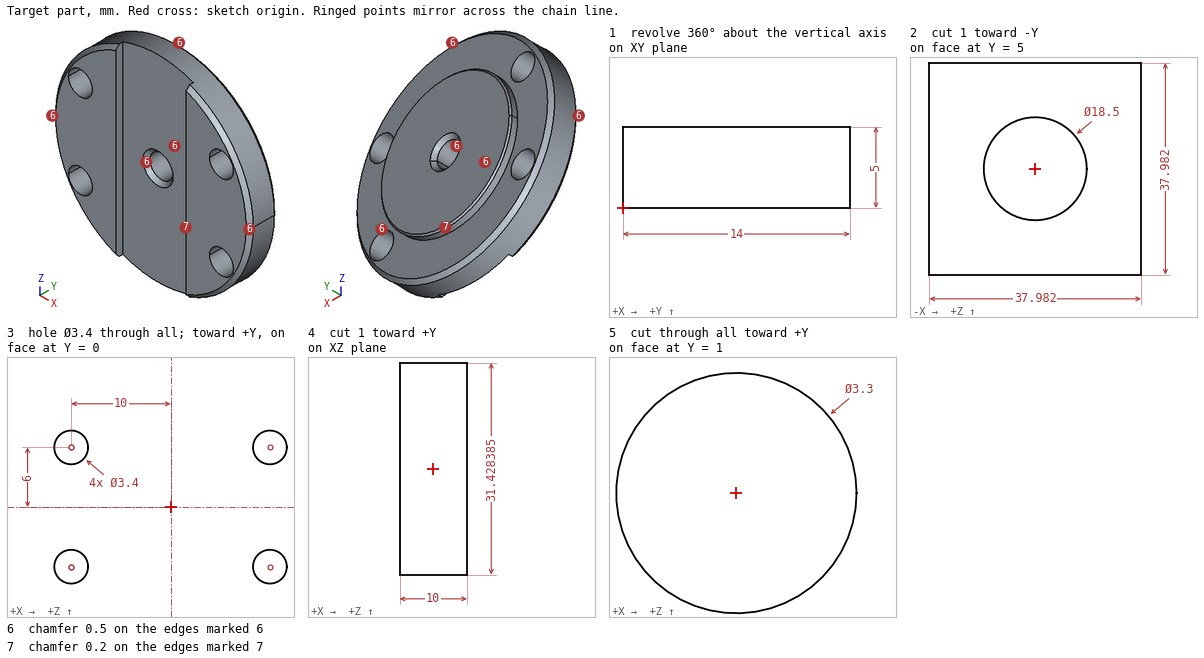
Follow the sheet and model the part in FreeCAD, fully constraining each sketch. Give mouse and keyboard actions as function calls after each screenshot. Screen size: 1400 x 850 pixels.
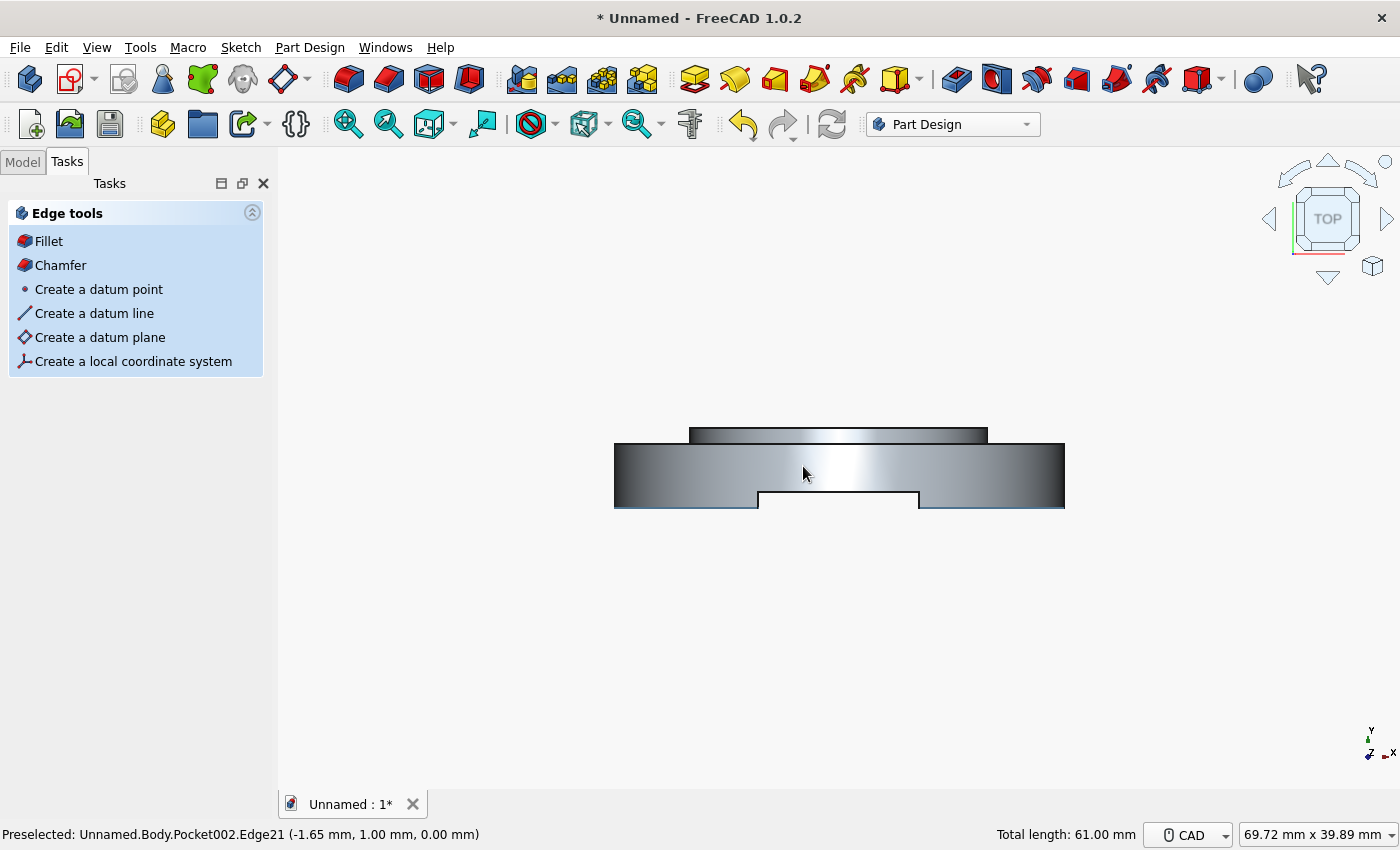
key(0)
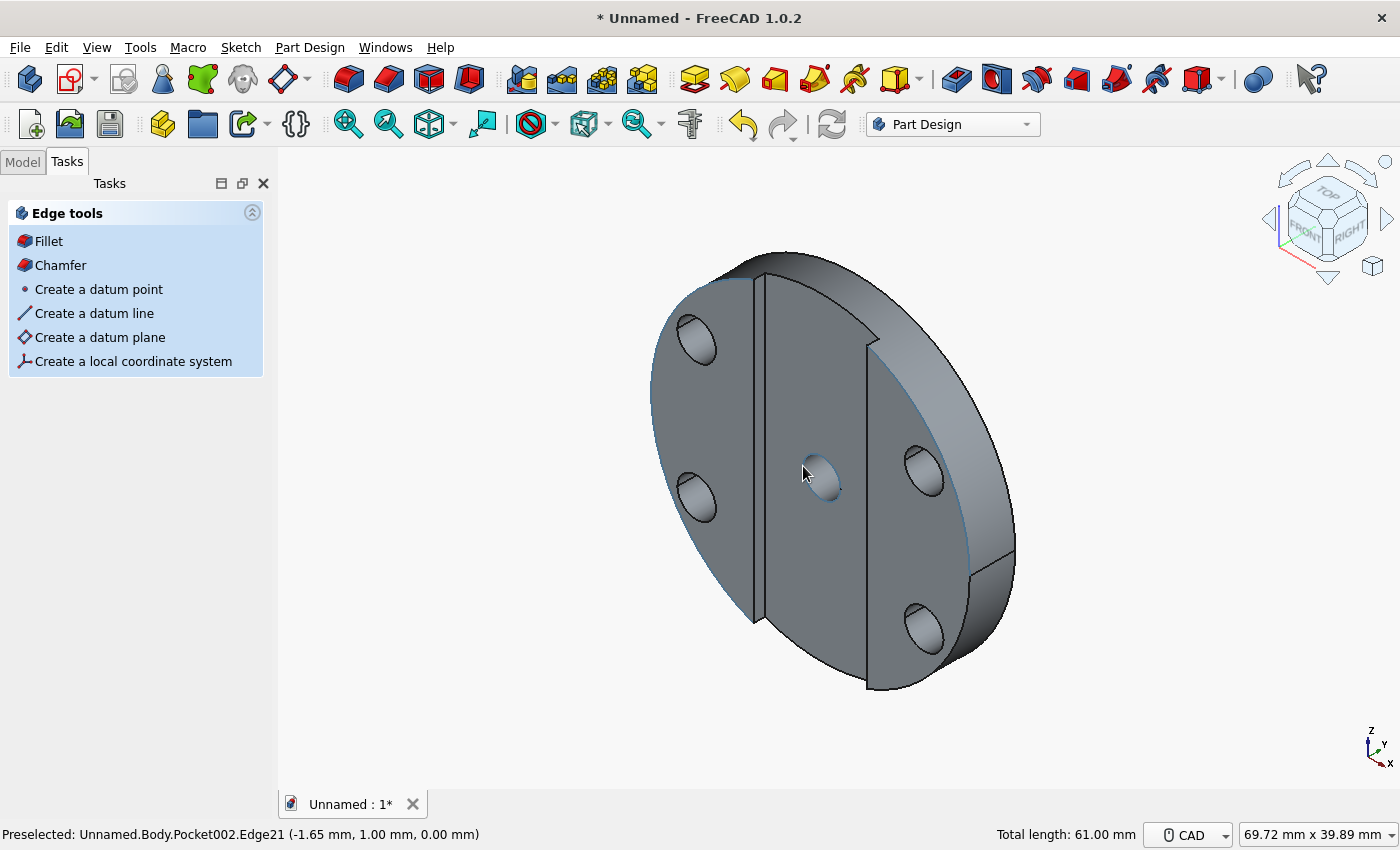
key(1)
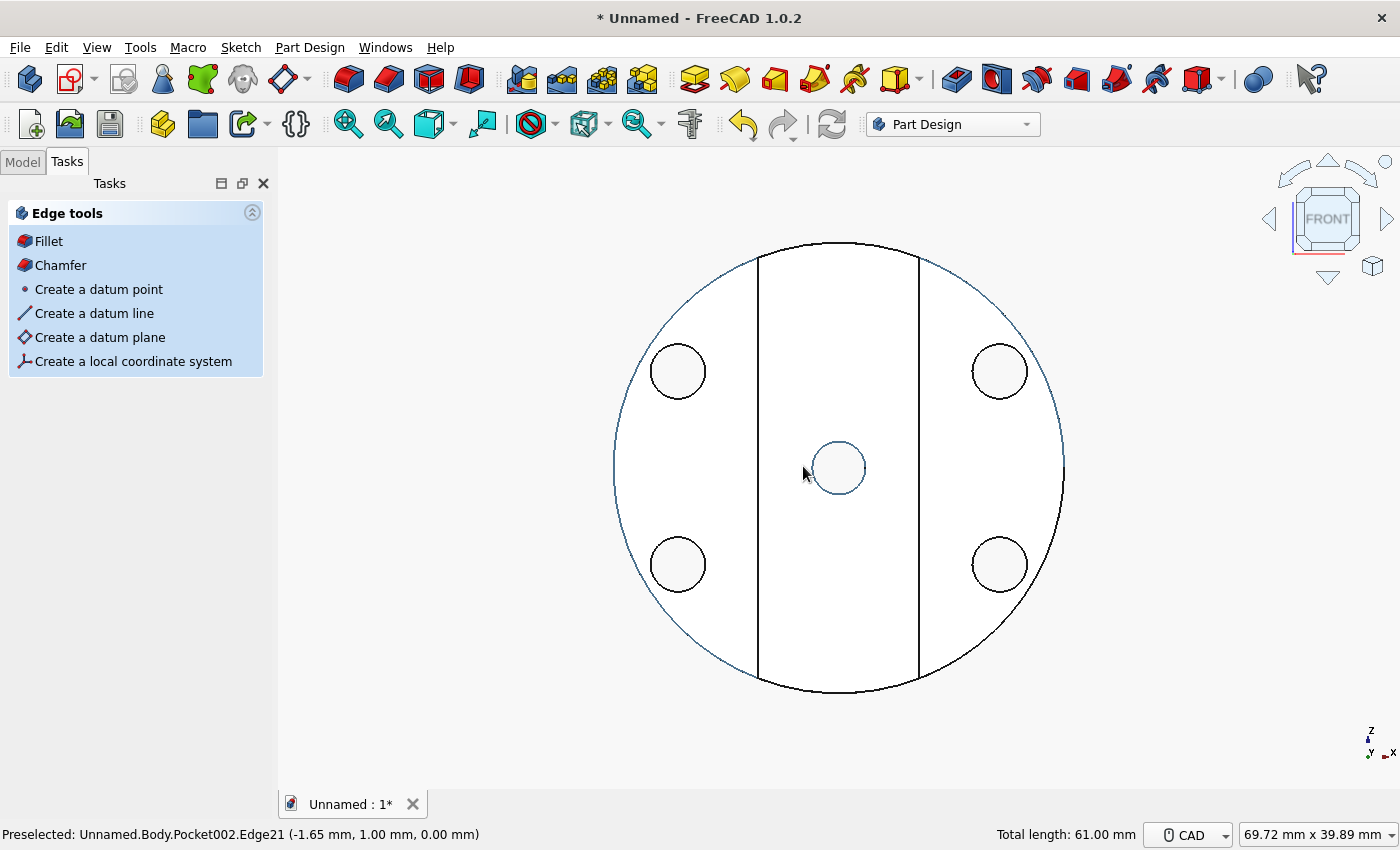
key(3)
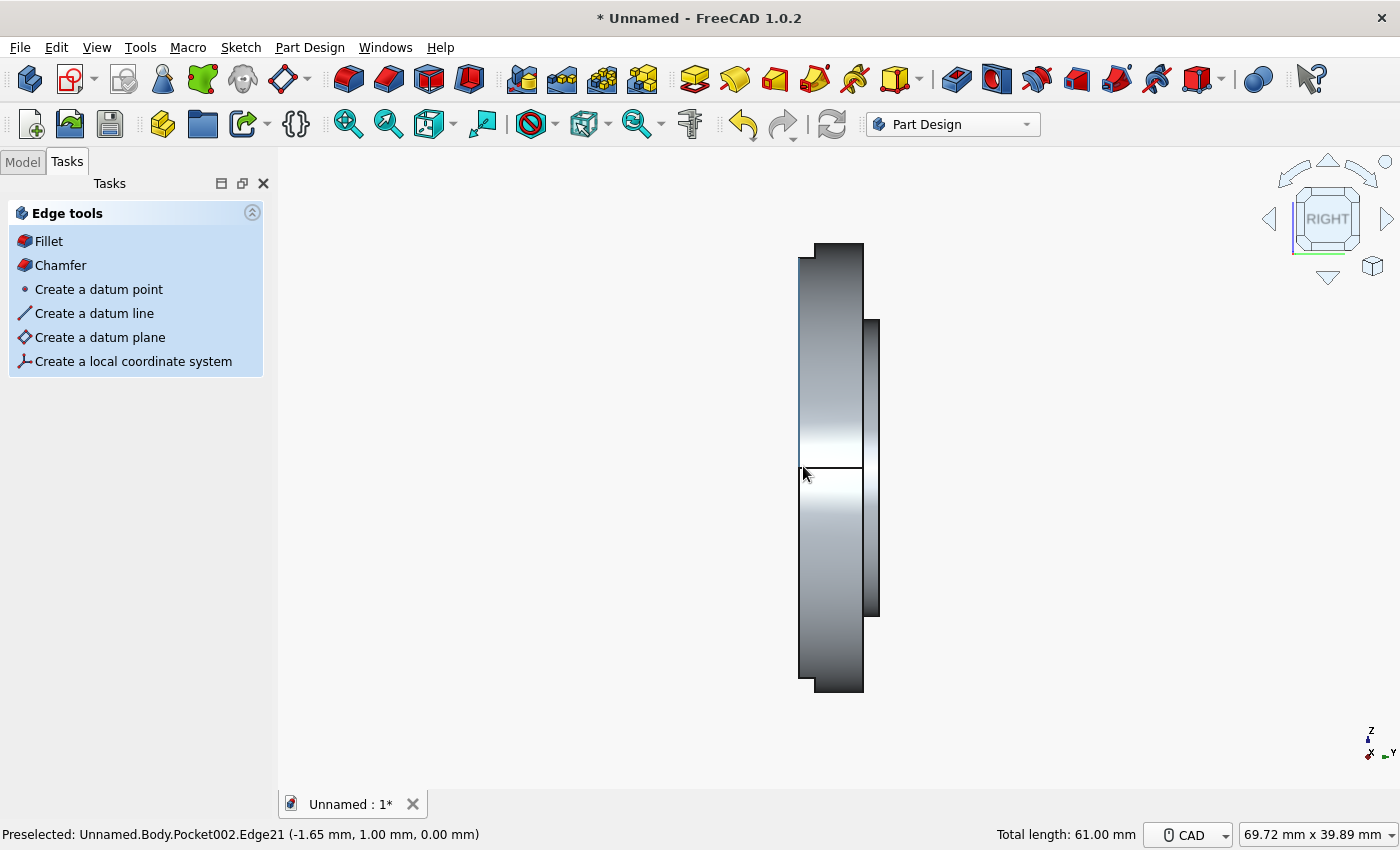
click(863, 621, ctrl)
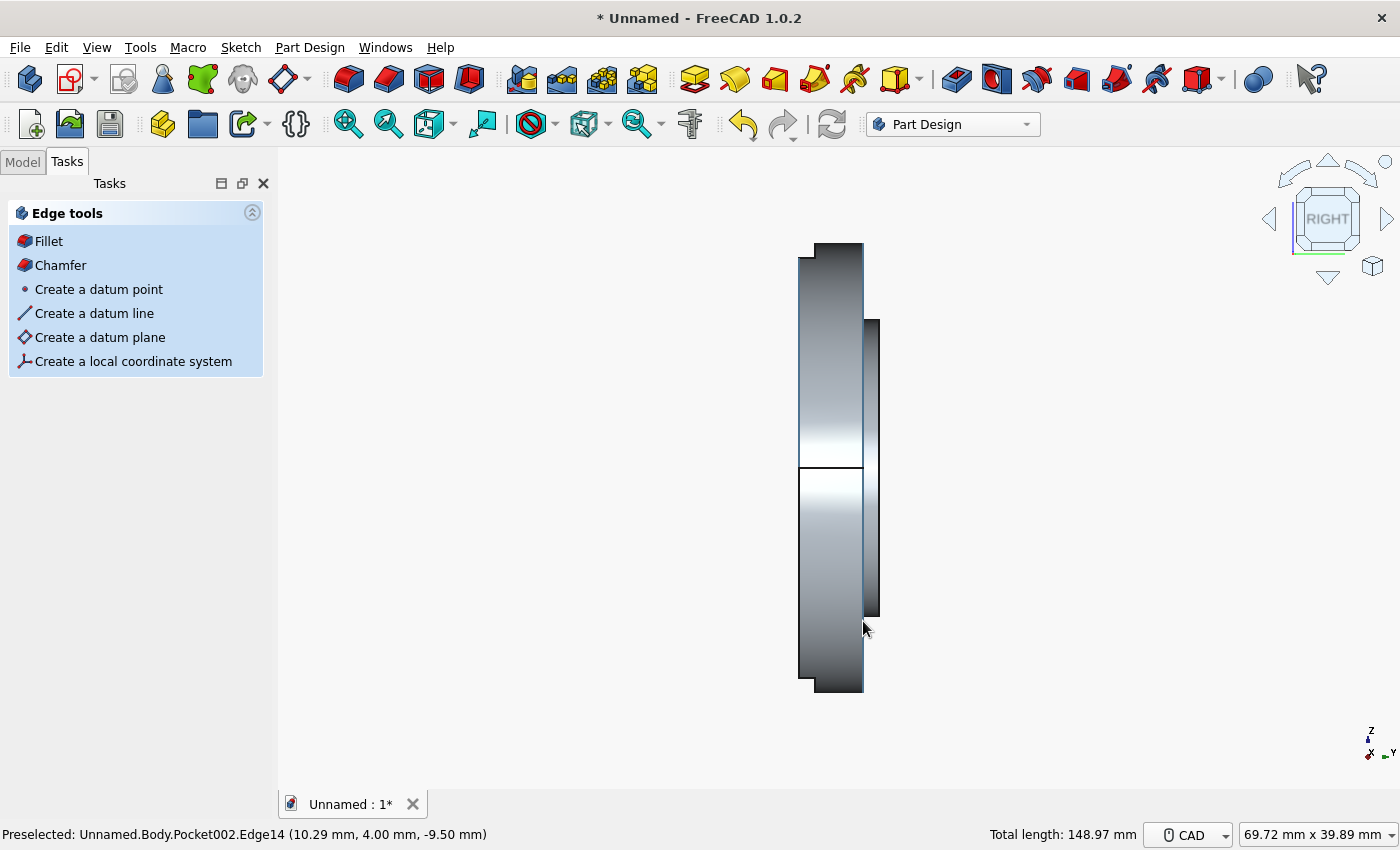
key(5)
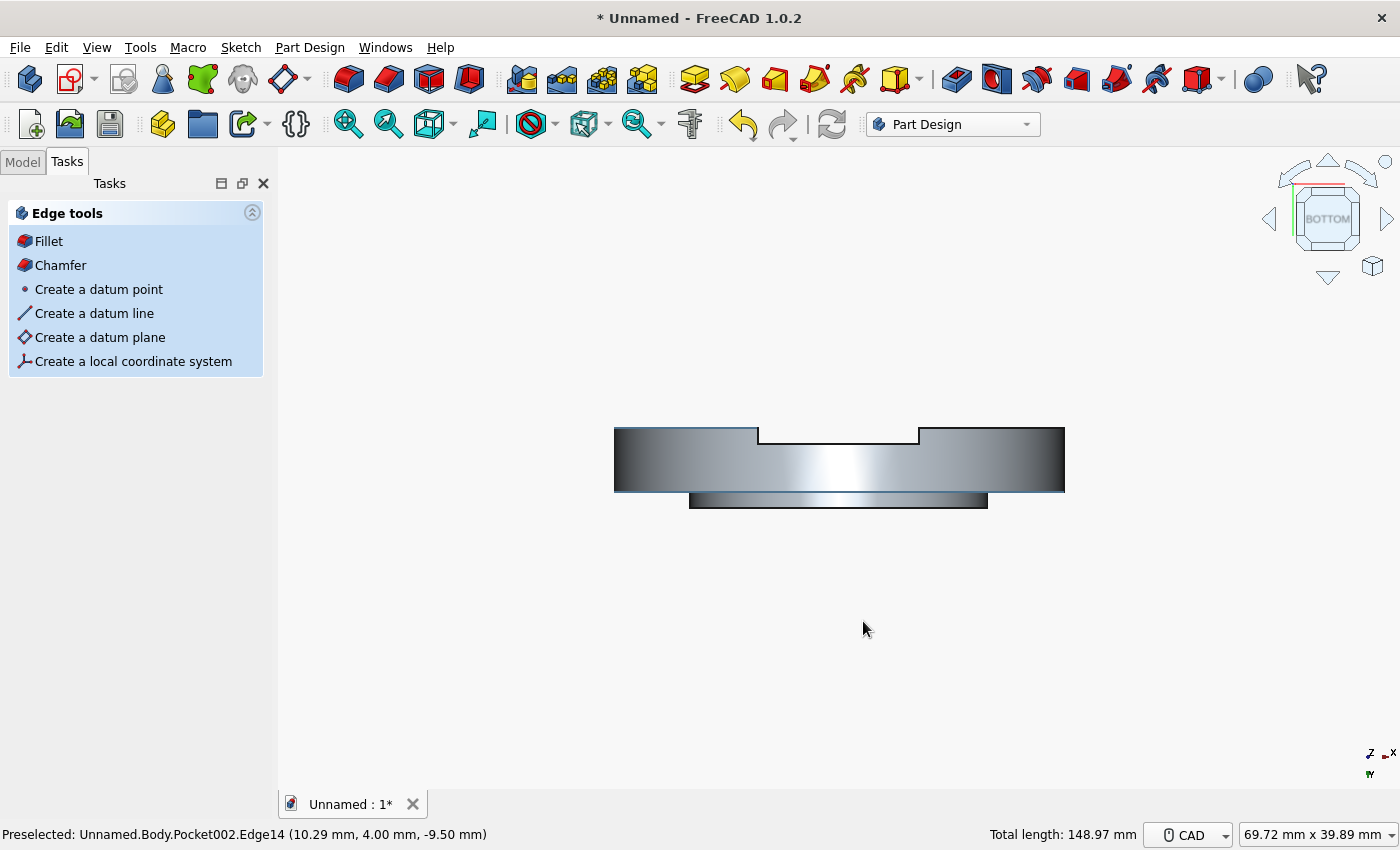
click(350, 124)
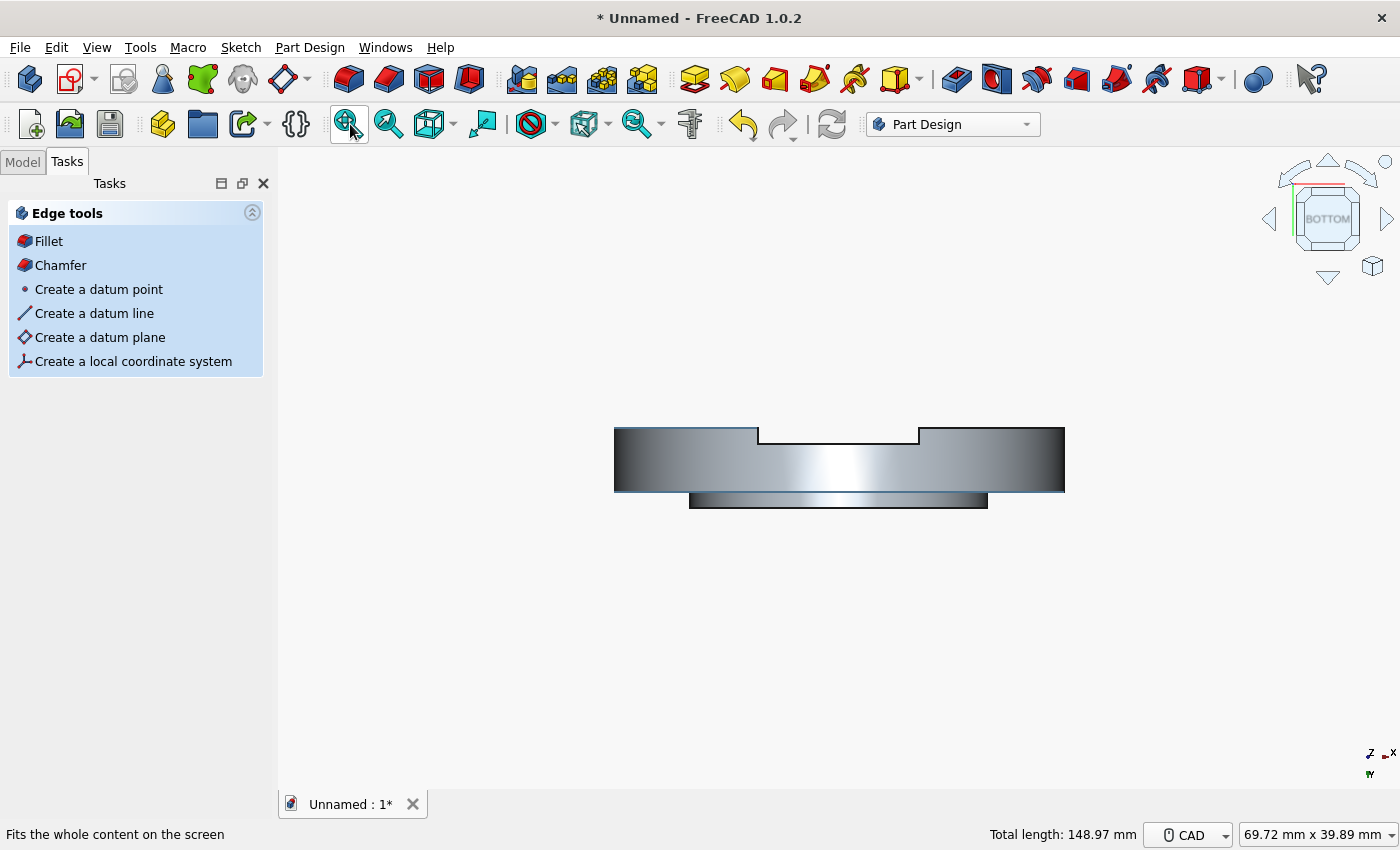
key(4)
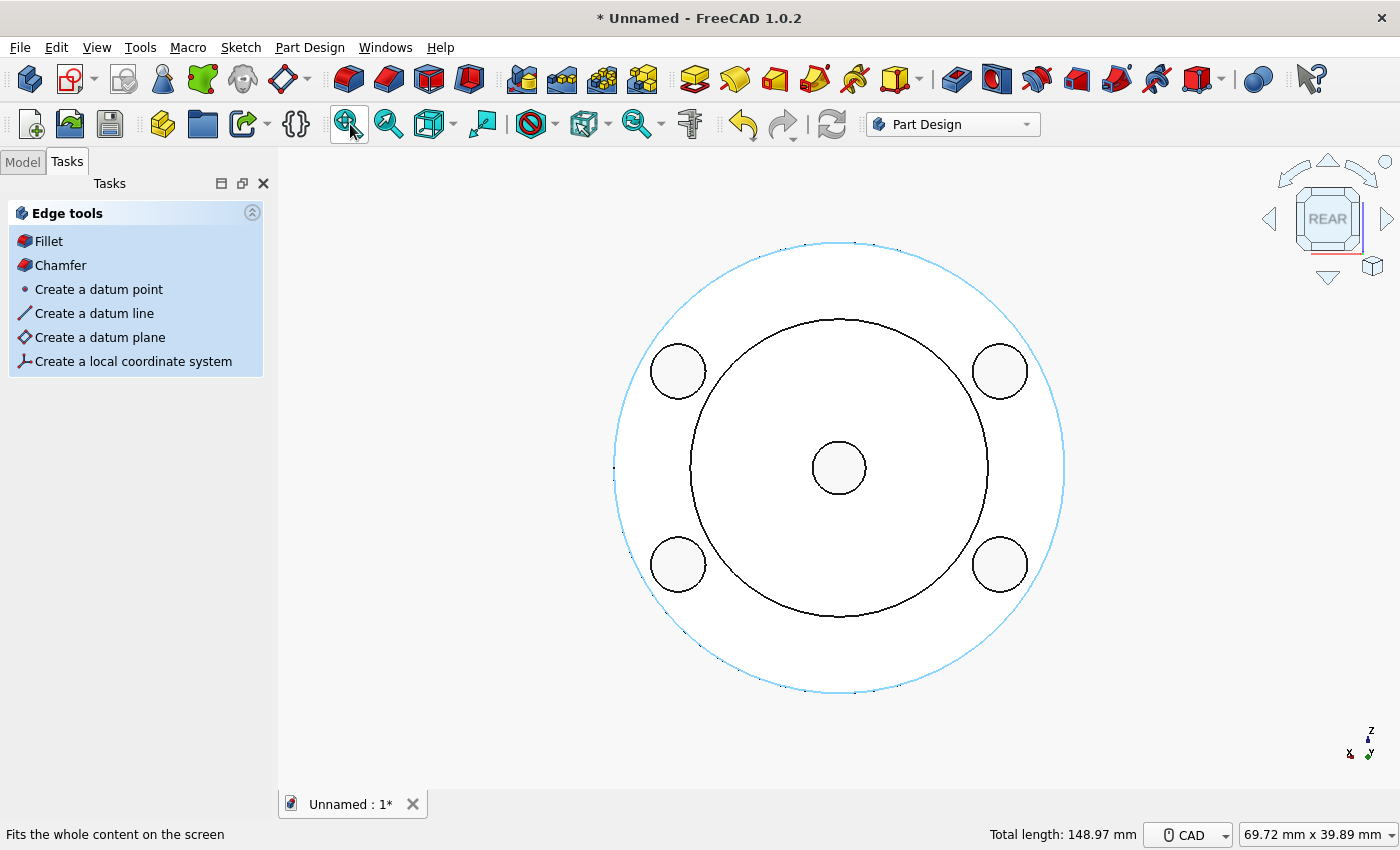
click(866, 467, ctrl)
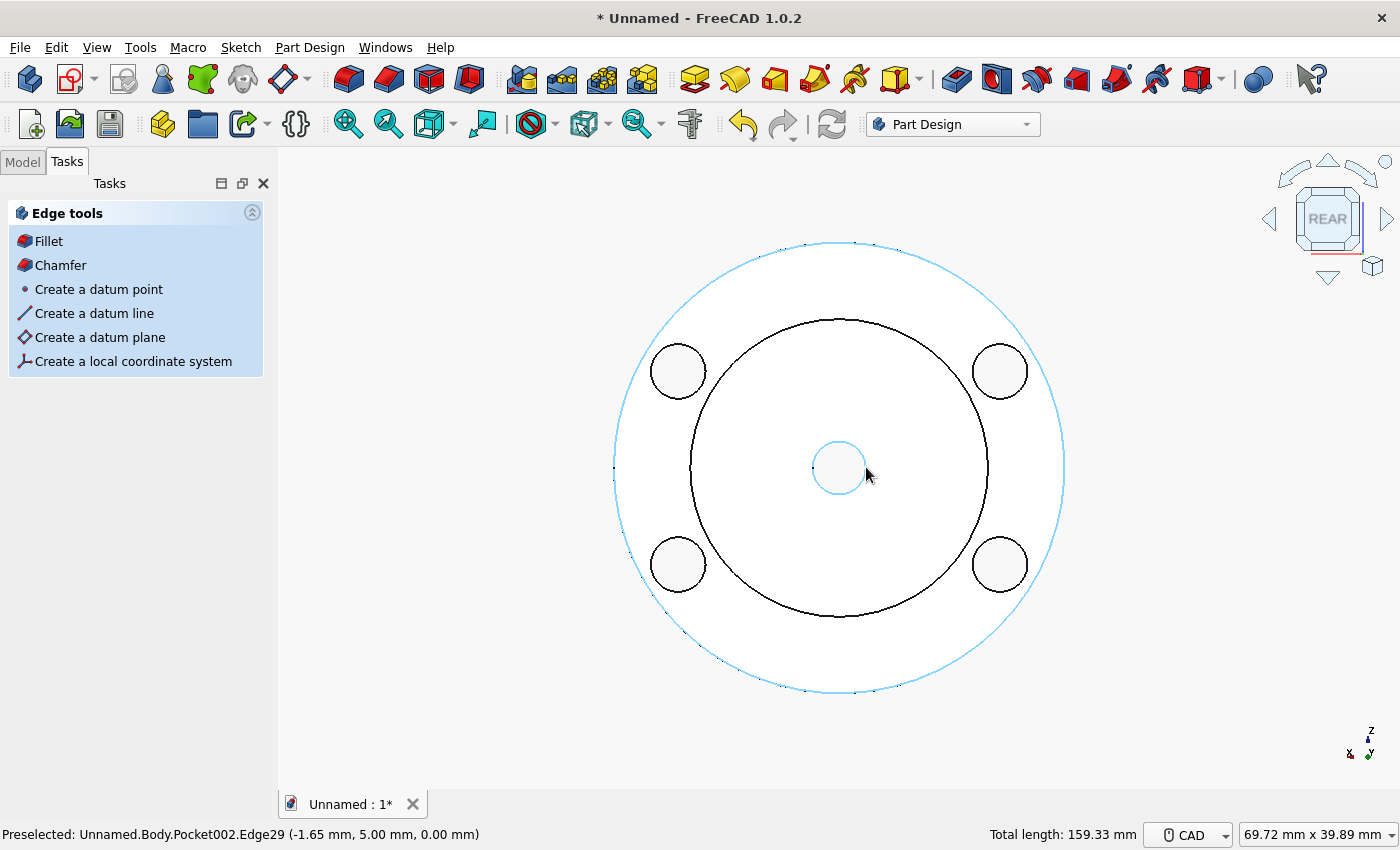
click(390, 80)